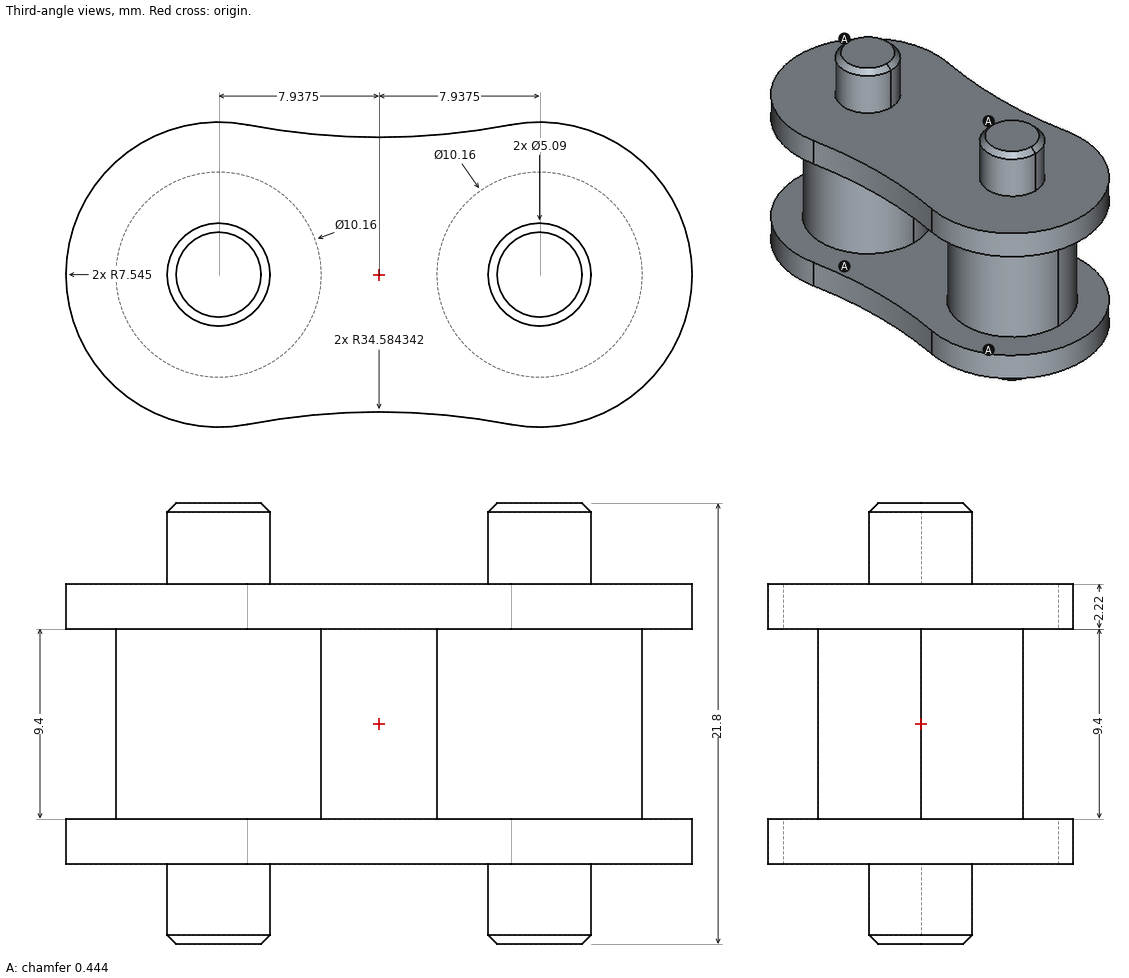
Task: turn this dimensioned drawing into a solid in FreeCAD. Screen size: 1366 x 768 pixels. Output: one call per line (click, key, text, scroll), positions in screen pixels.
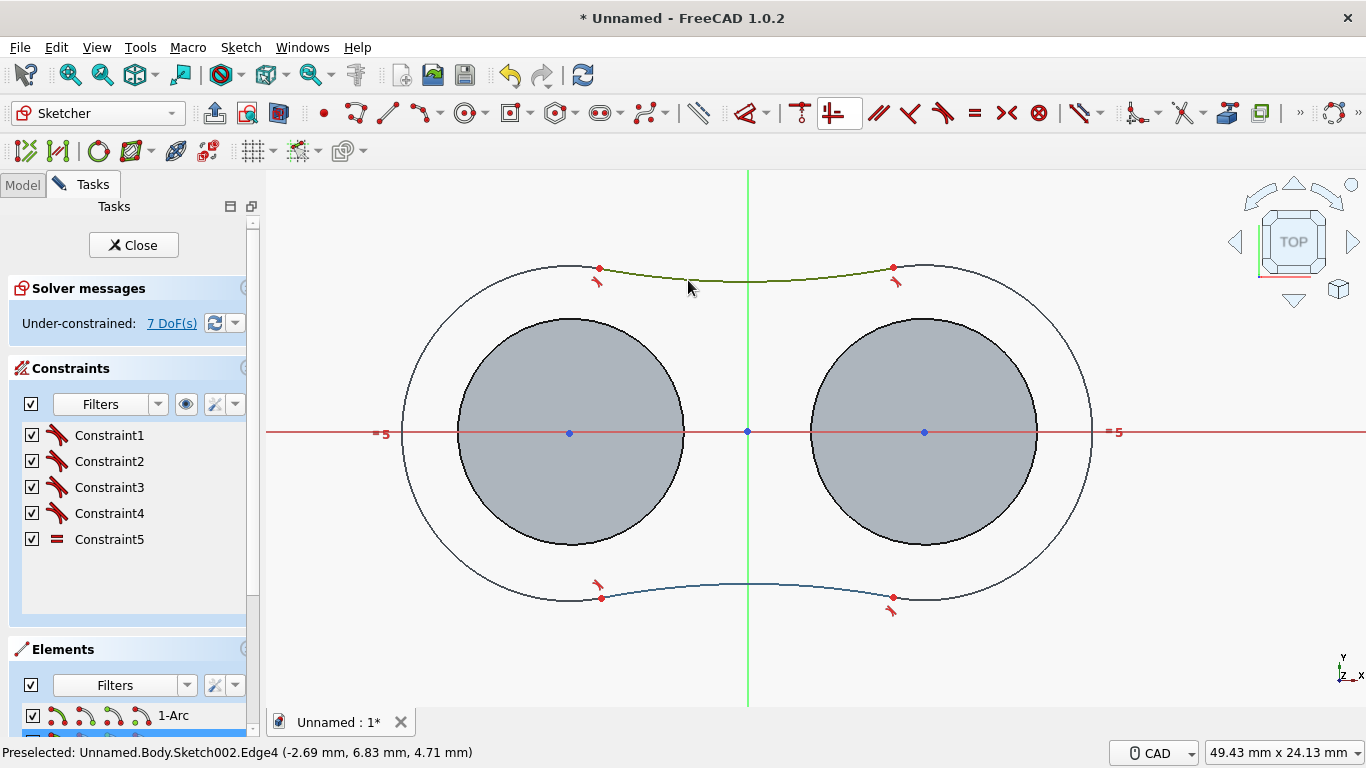
click(976, 114)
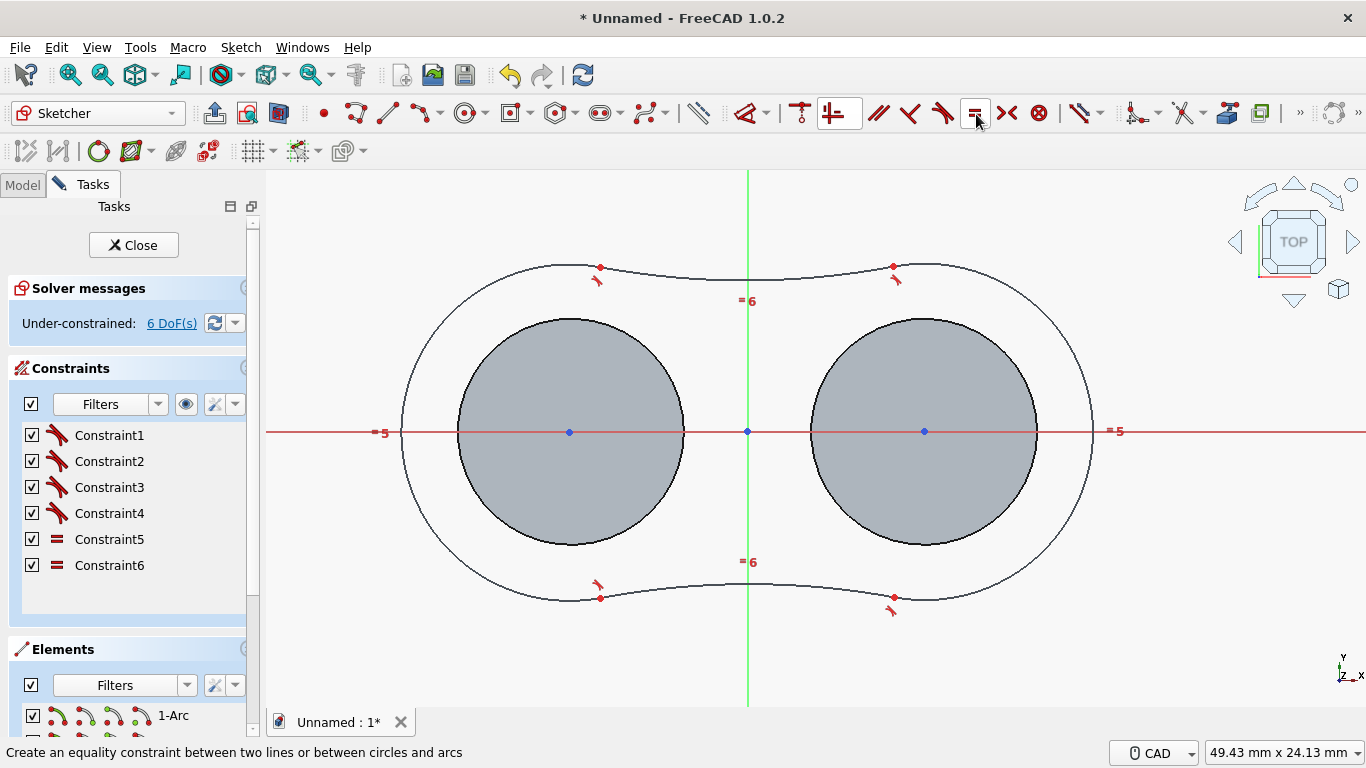
click(570, 433)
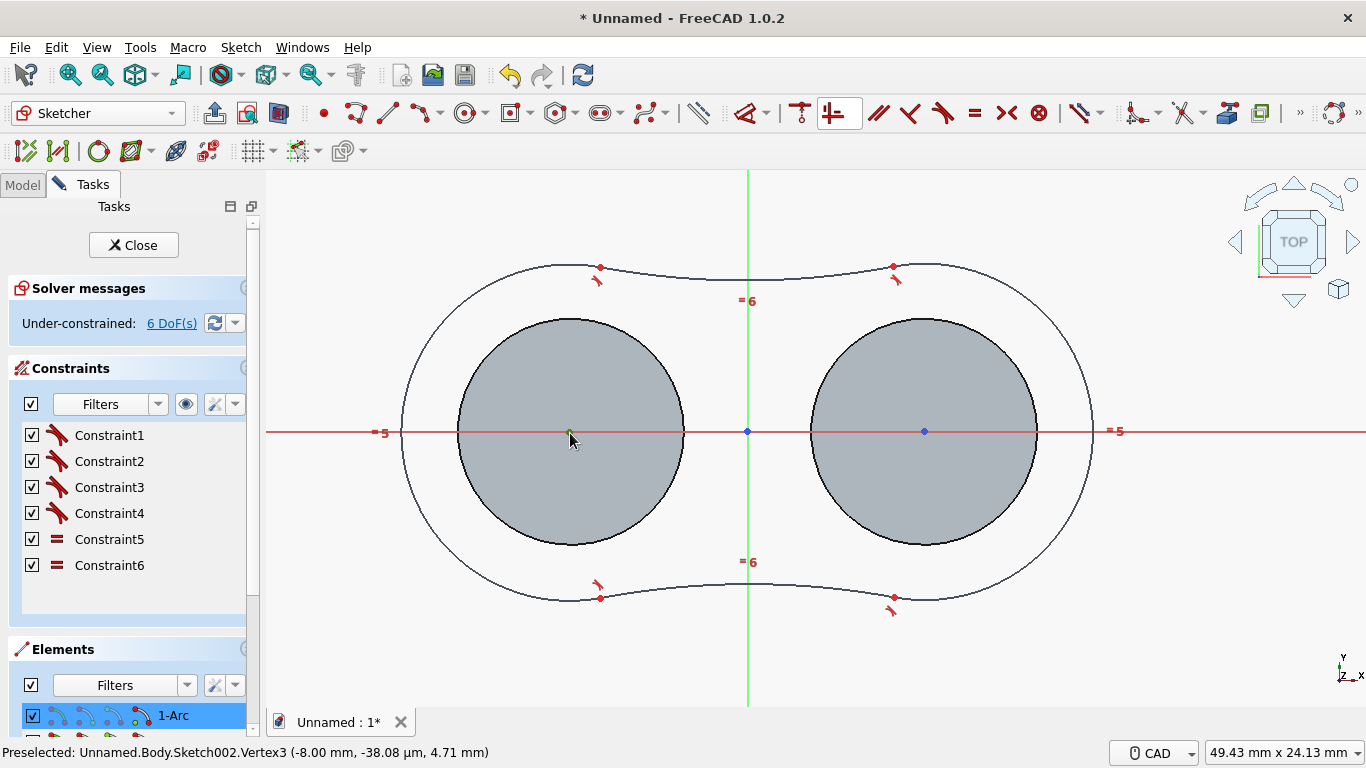
click(359, 432)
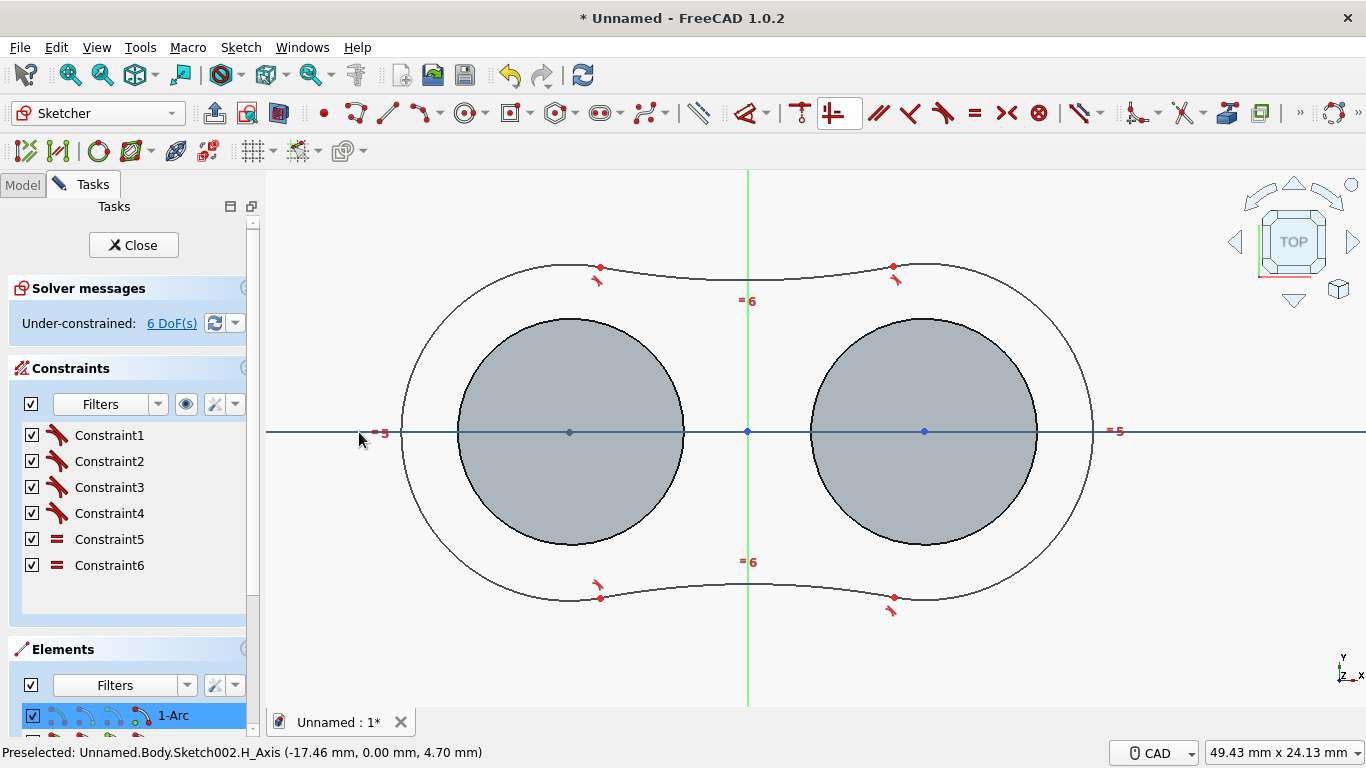
key(c)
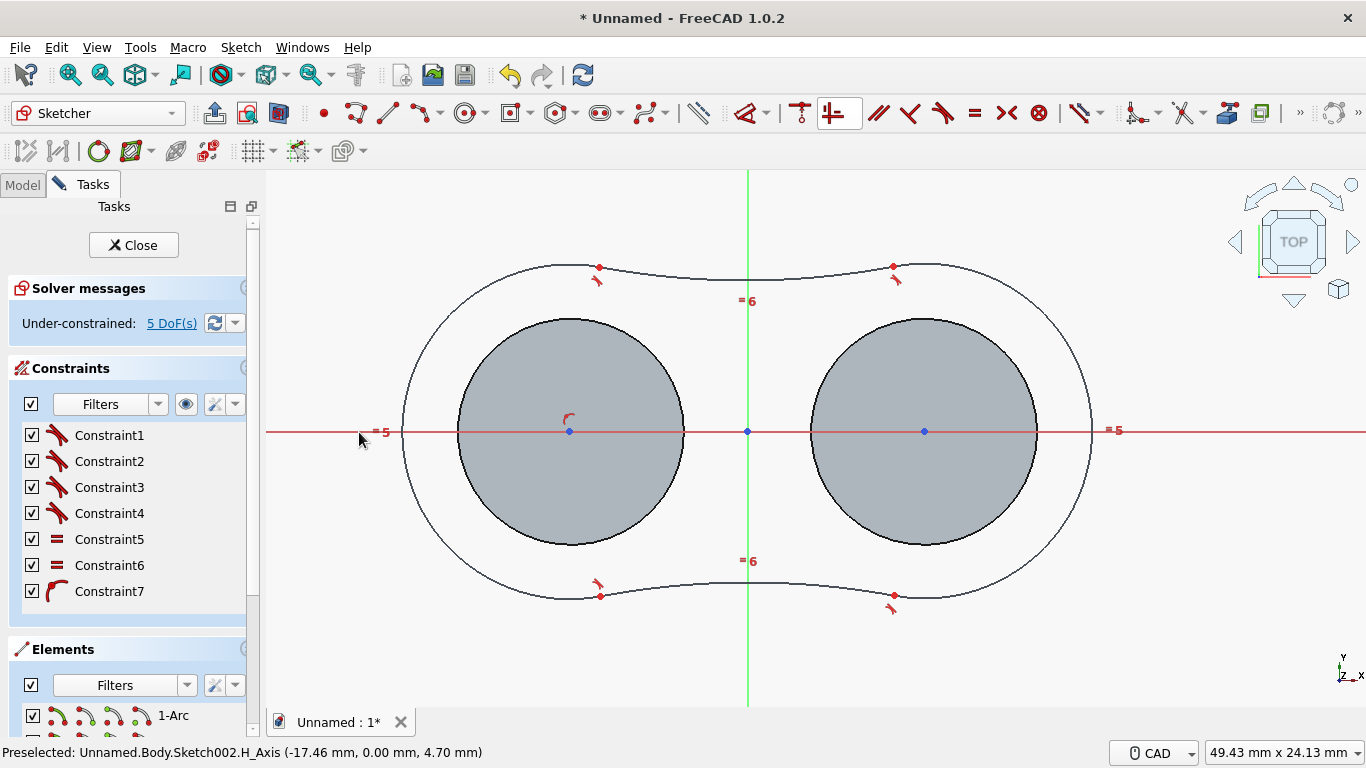
scroll(747, 271, down, 6)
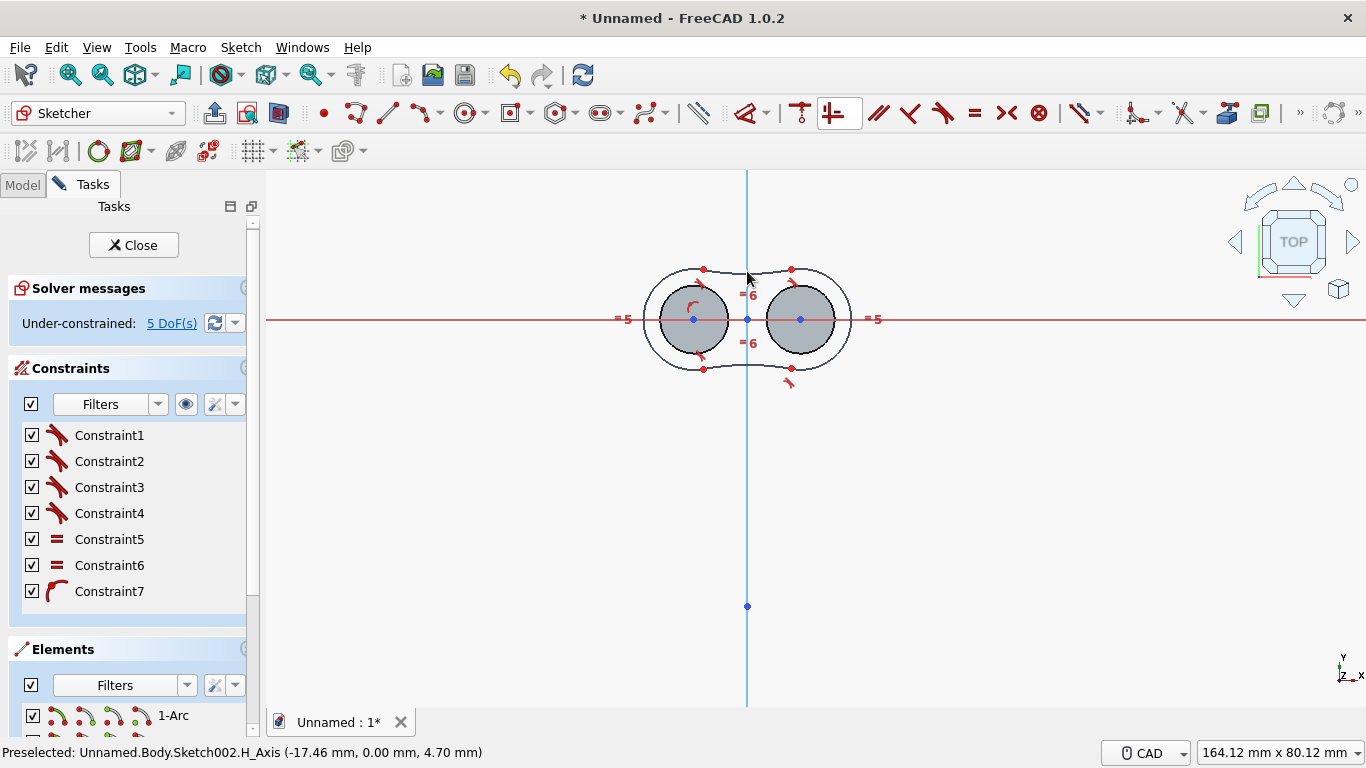
click(748, 607)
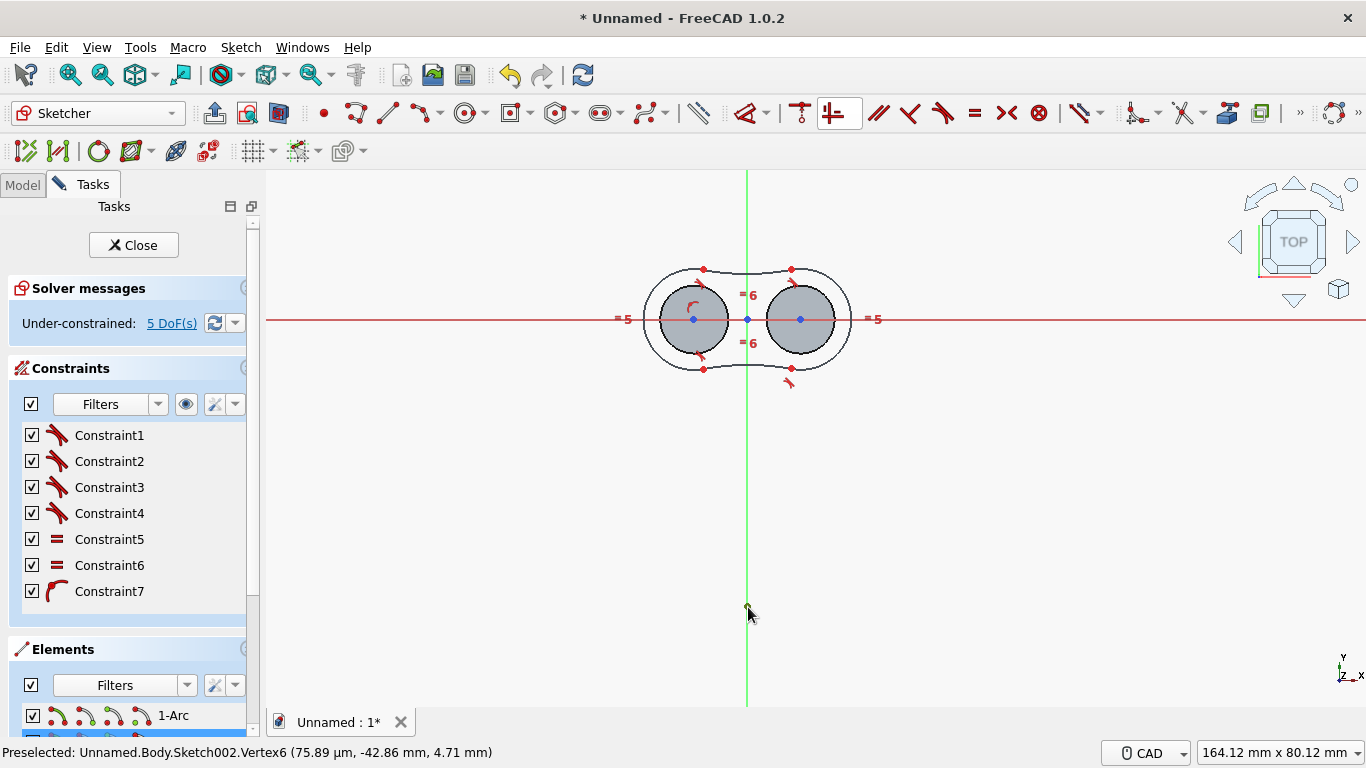
click(747, 645)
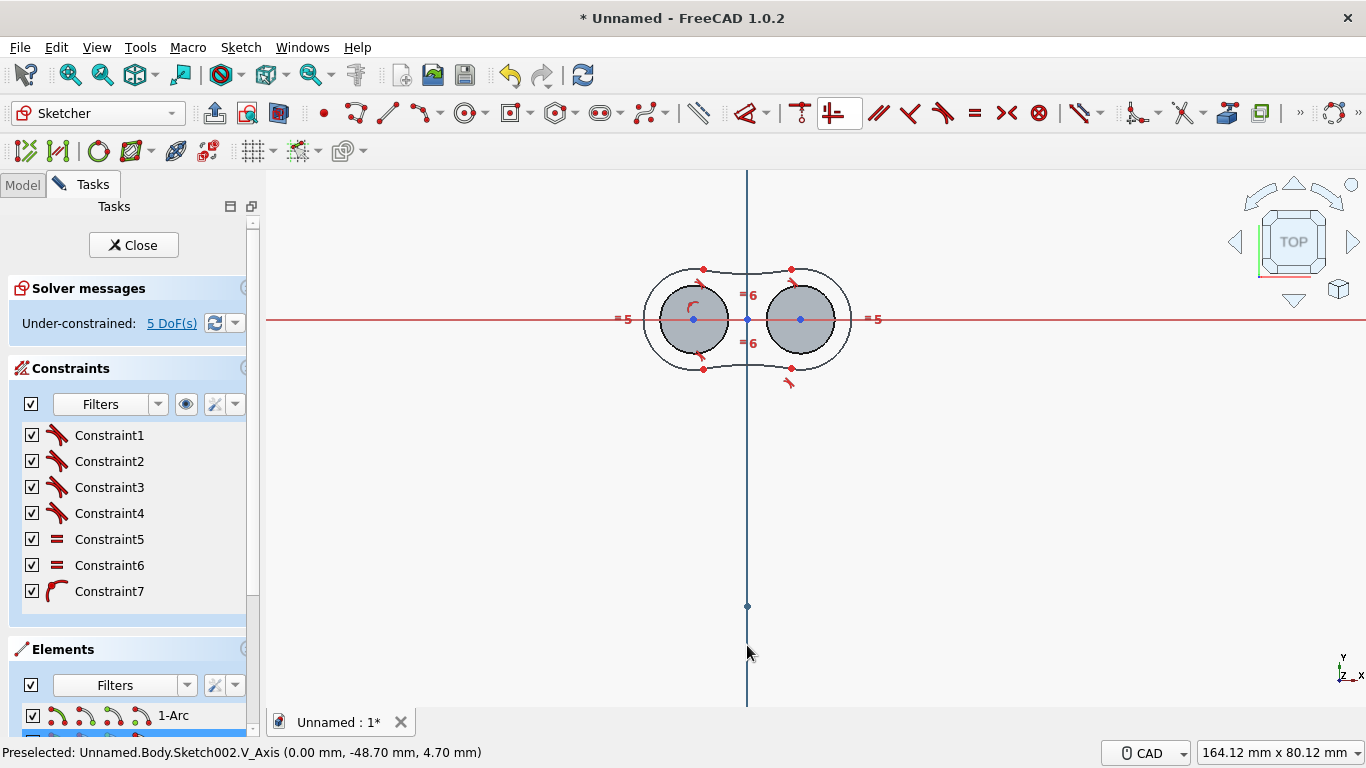
click(800, 114)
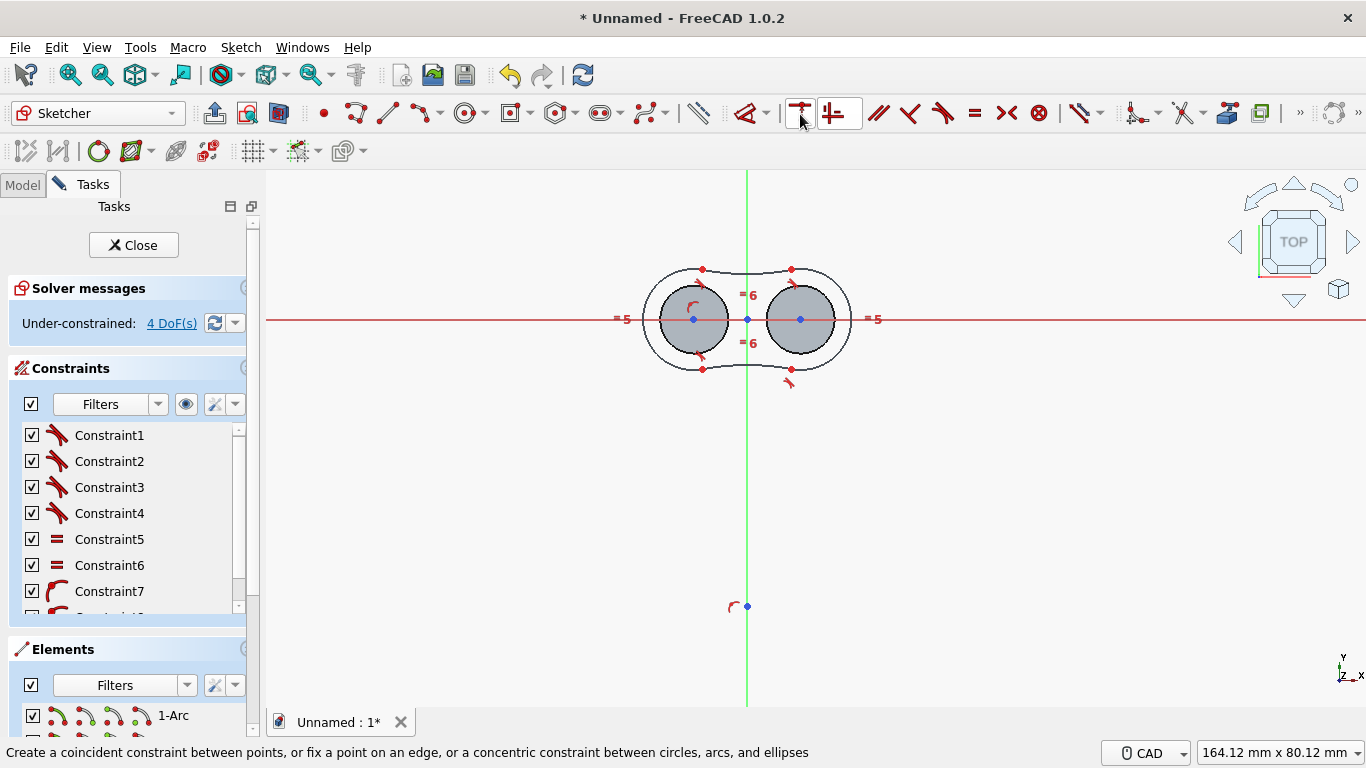
click(801, 319)